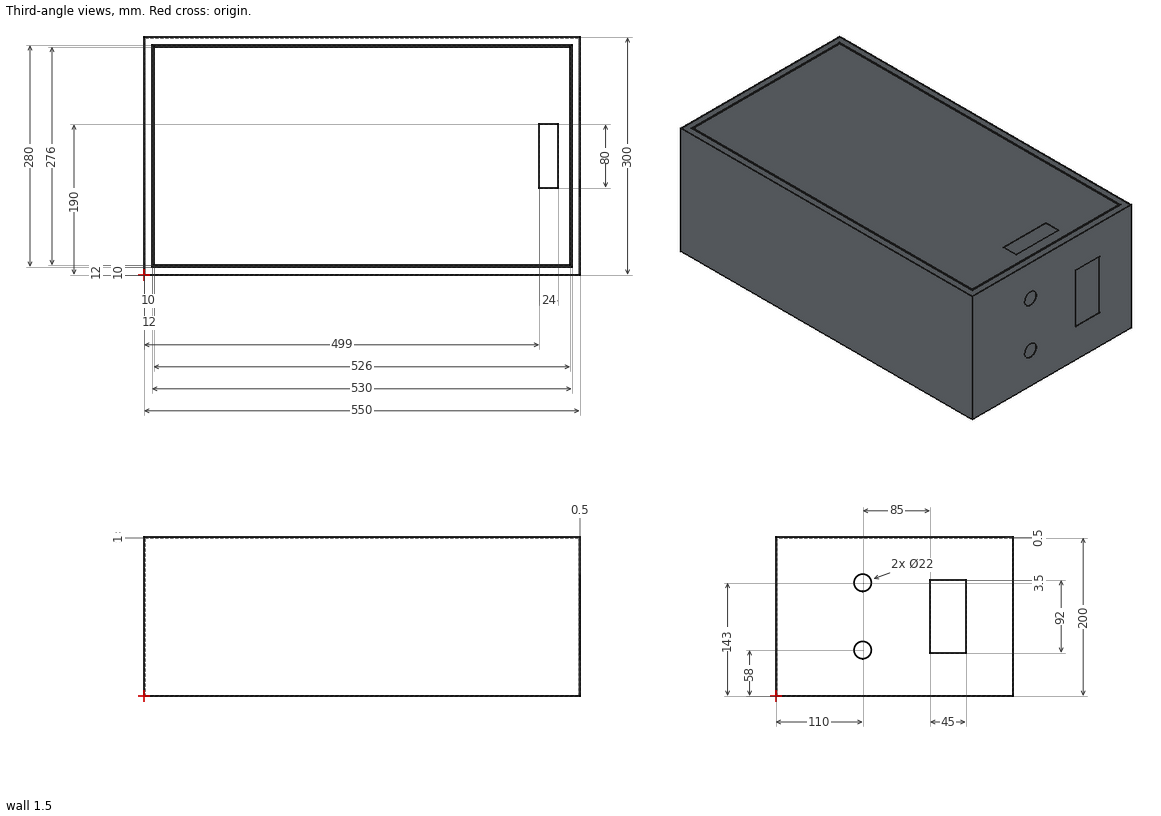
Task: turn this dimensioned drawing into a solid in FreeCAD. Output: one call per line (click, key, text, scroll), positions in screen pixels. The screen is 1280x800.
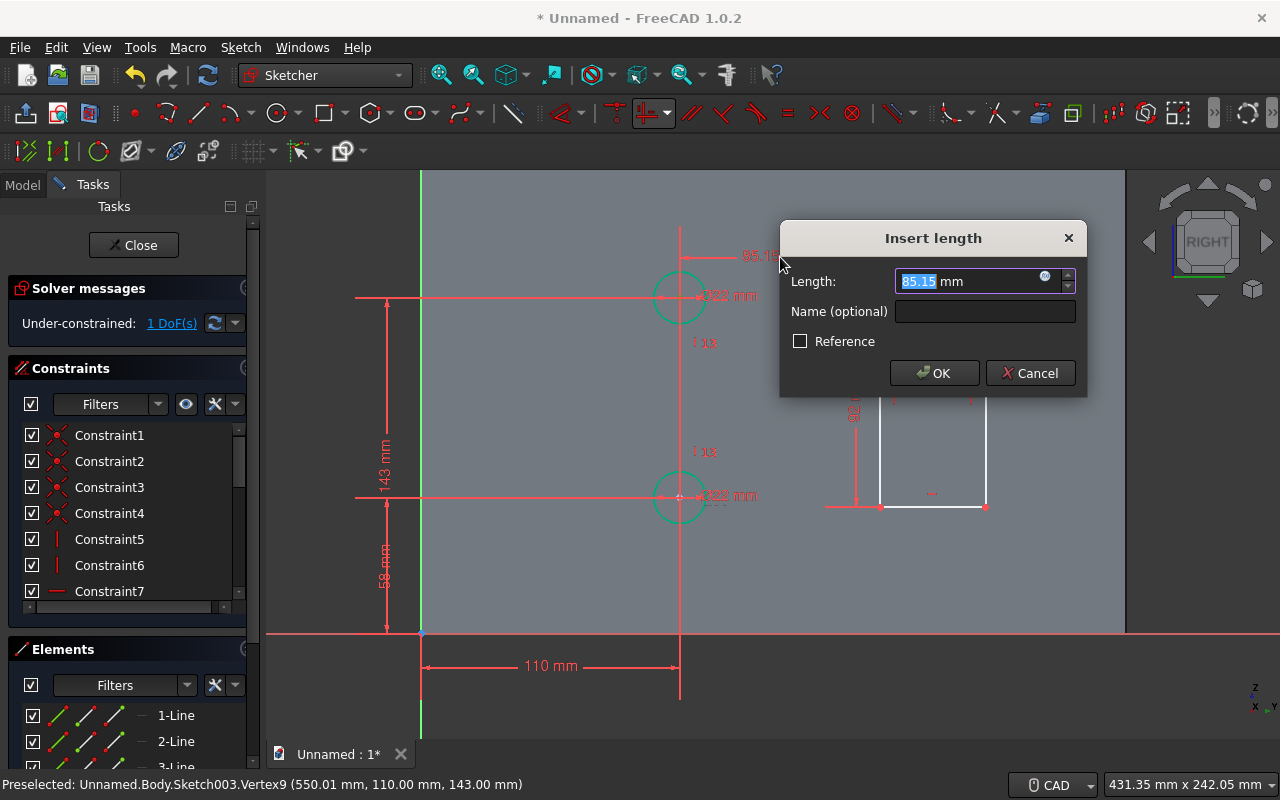
text(85)
key(Return)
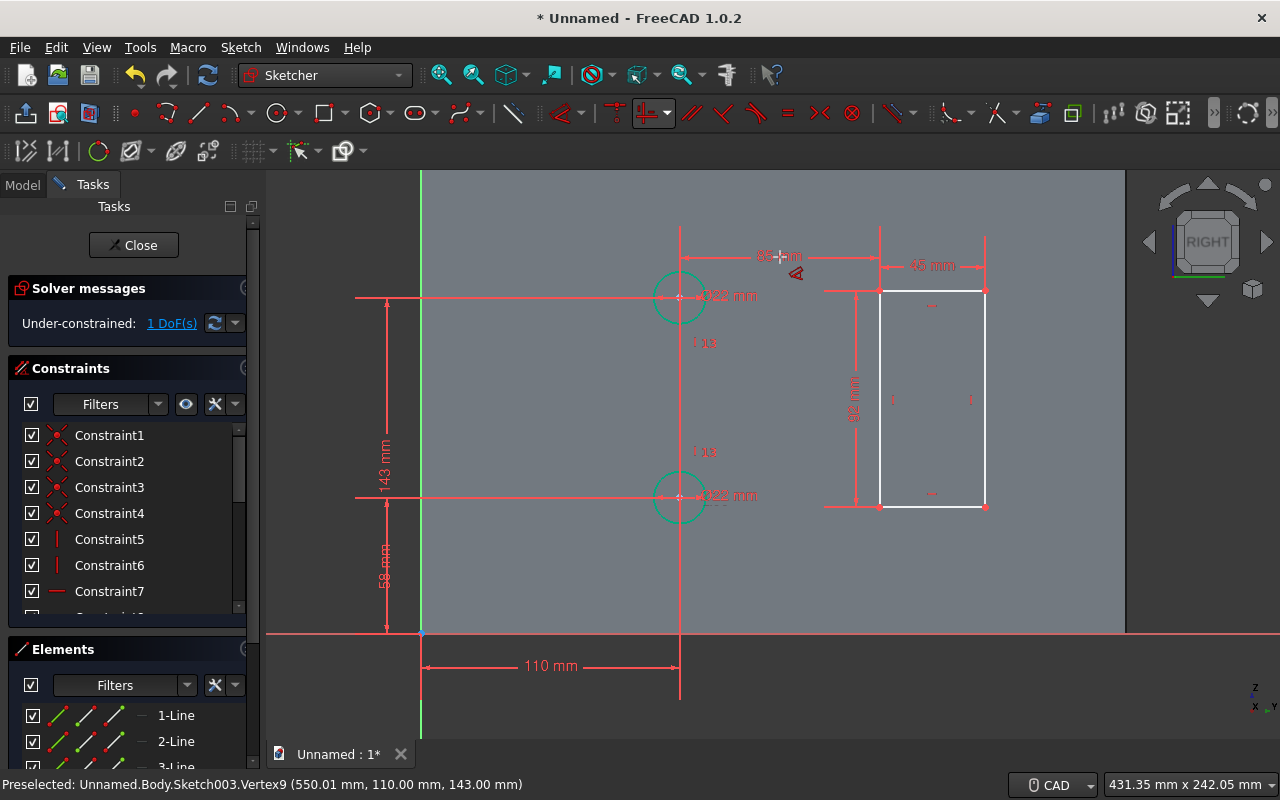
scroll(880, 291, up, 8)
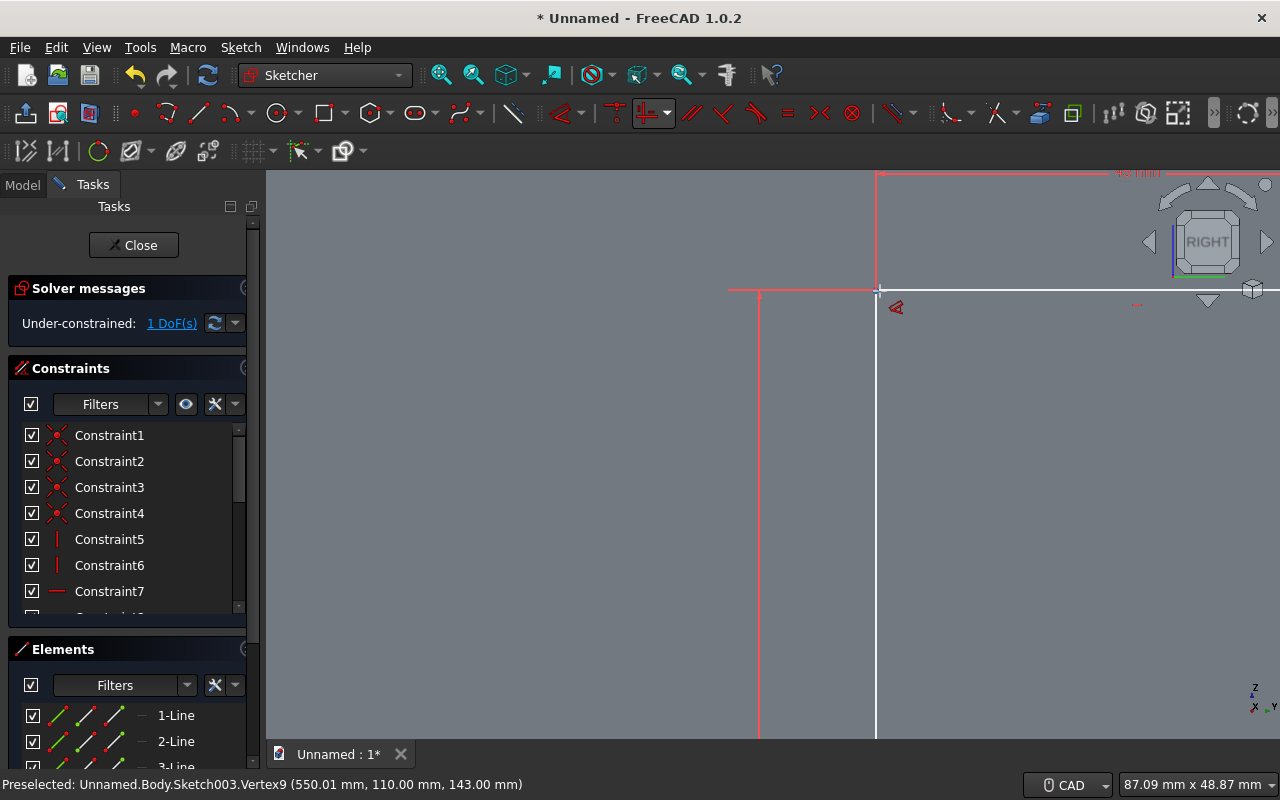
click(876, 290)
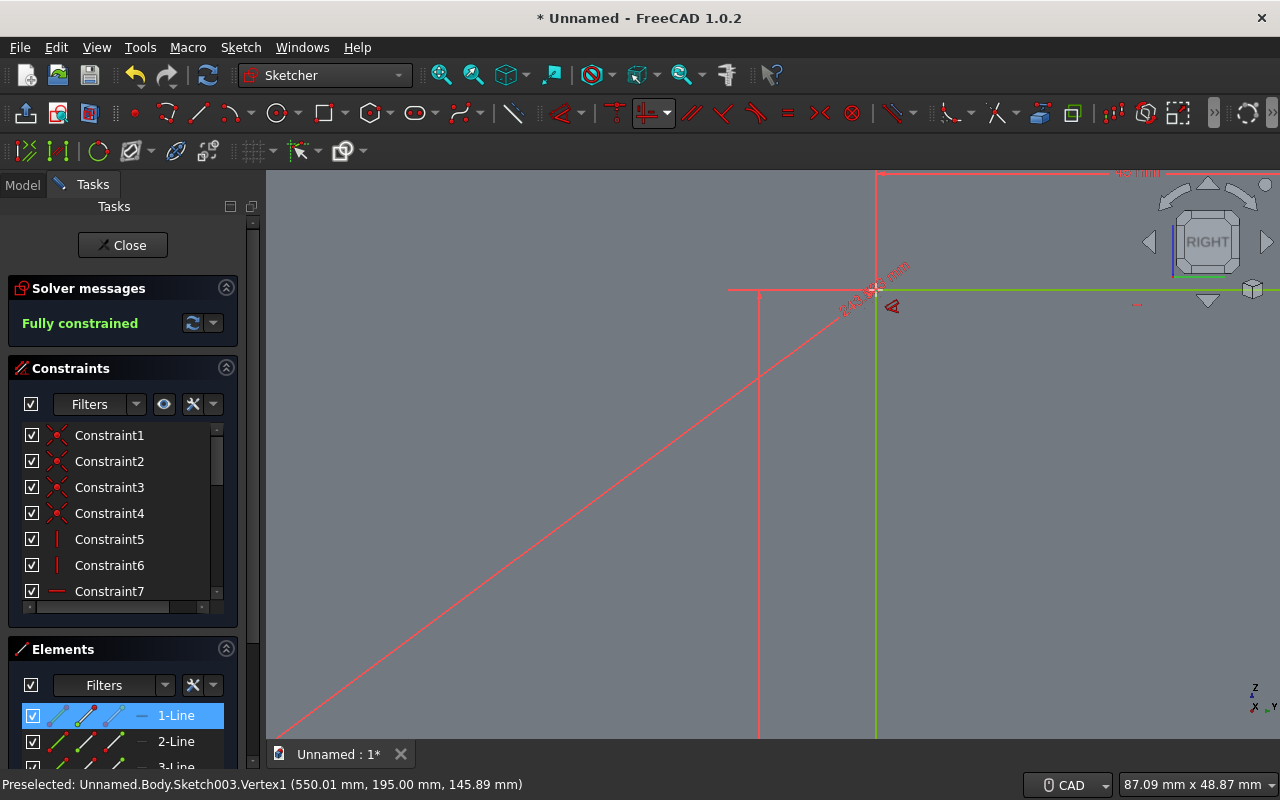
scroll(882, 293, down, 8)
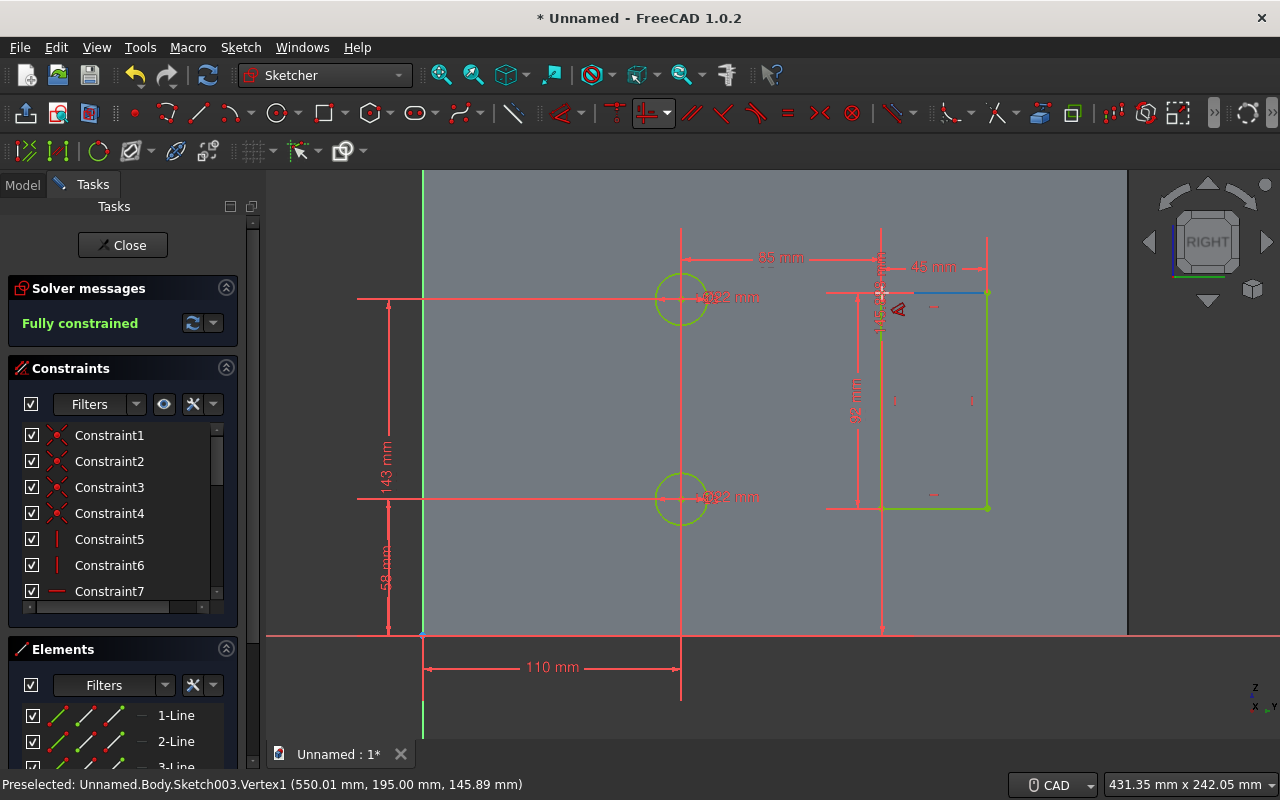
scroll(681, 299, up, 8)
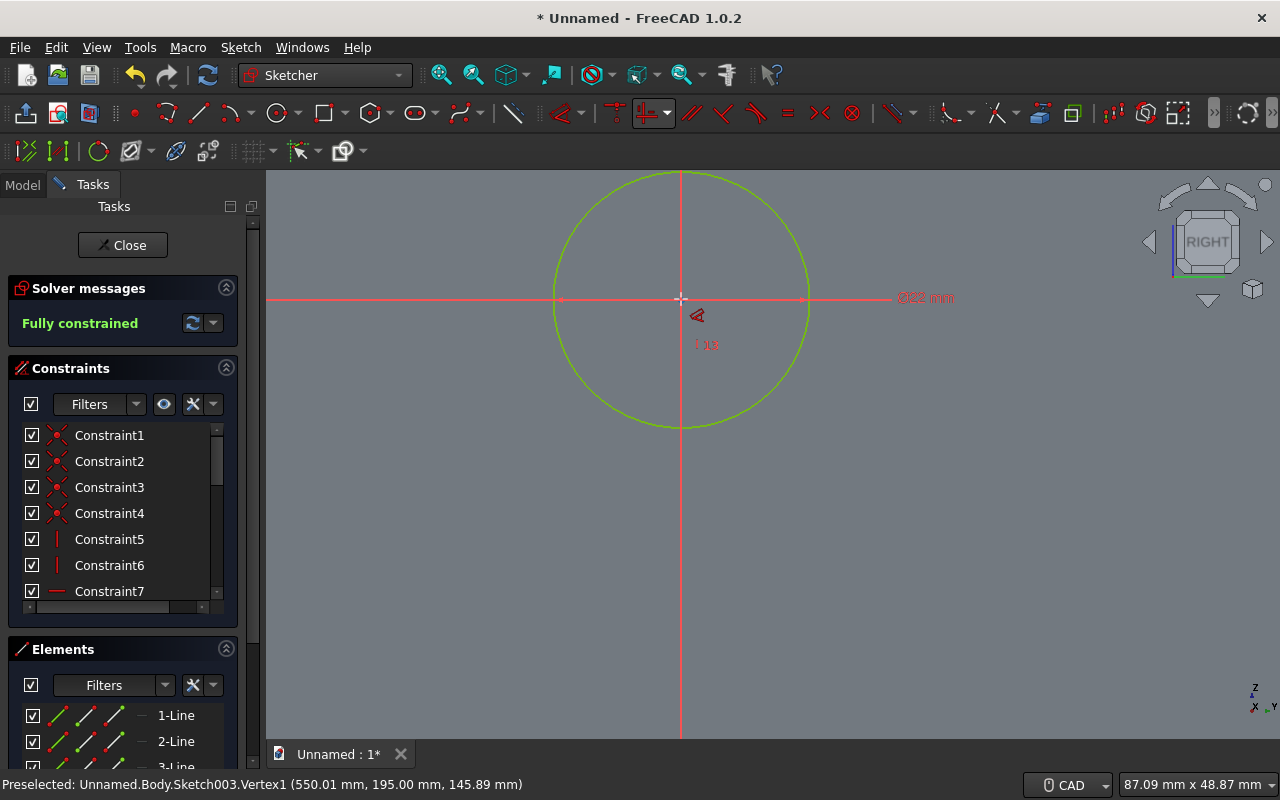
click(681, 300)
click(647, 283)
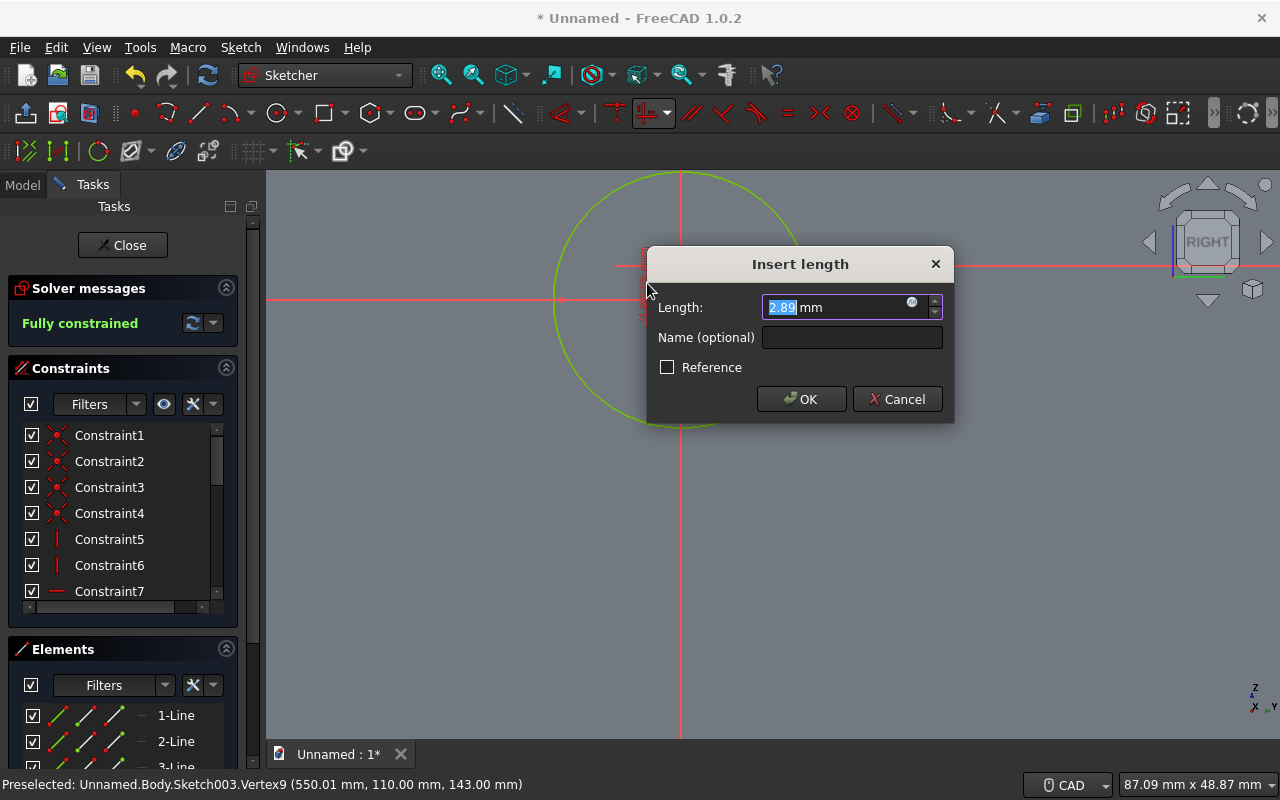
text(3.5)
key(Return)
key(Escape)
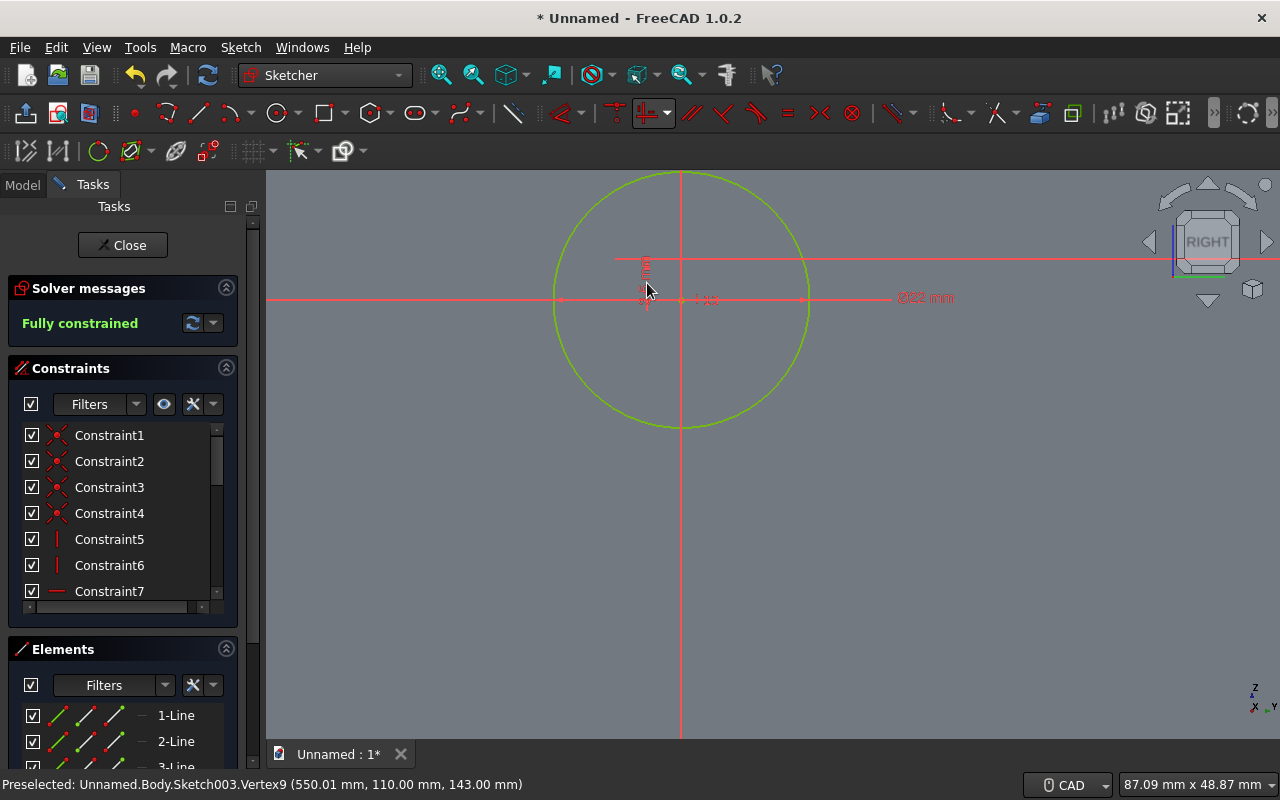
click(123, 245)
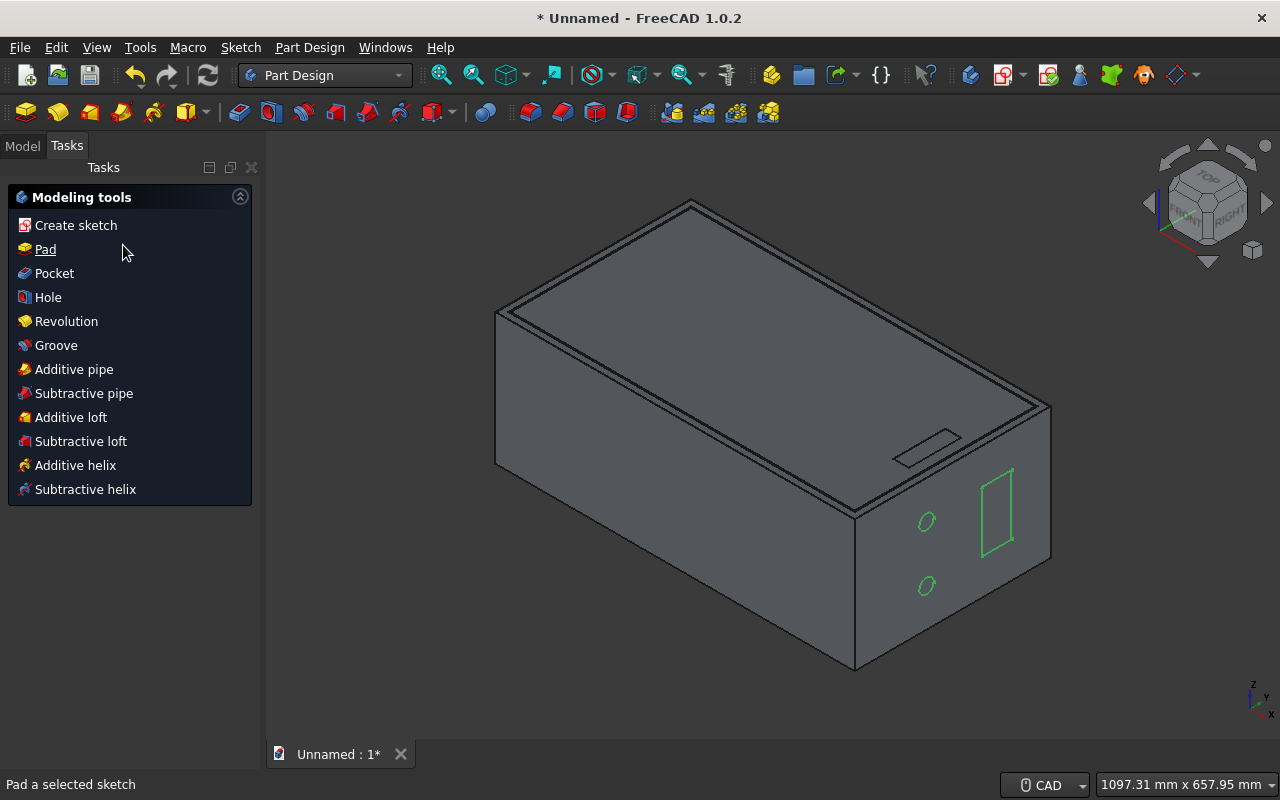
click(240, 112)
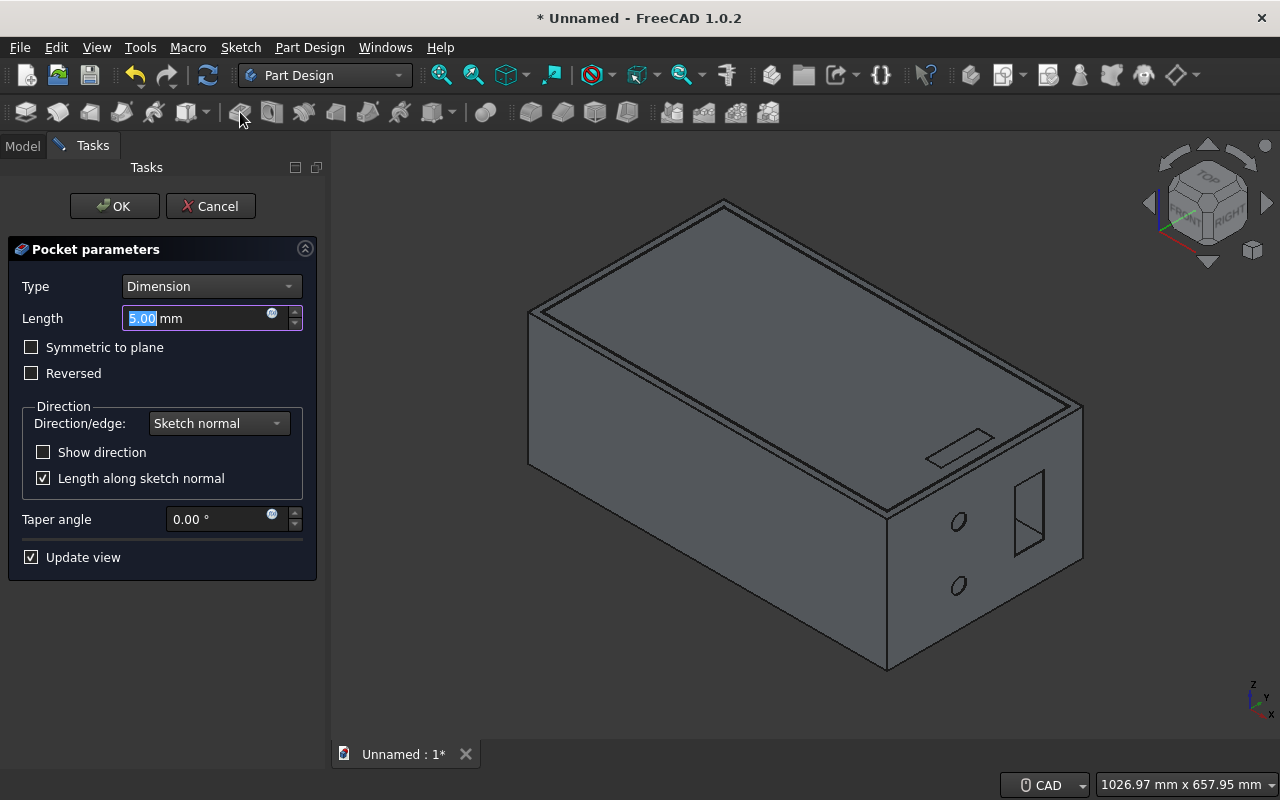
text(0.5)
key(Tab)